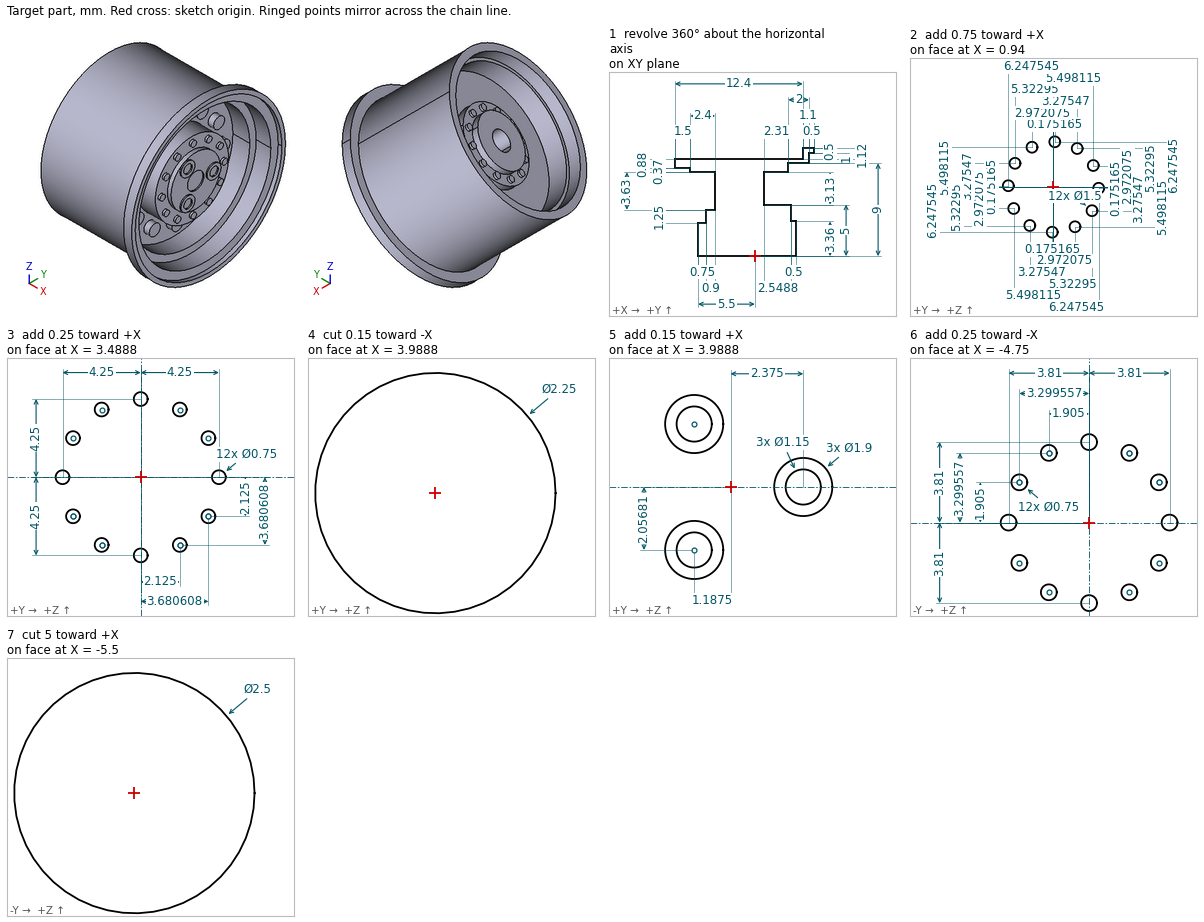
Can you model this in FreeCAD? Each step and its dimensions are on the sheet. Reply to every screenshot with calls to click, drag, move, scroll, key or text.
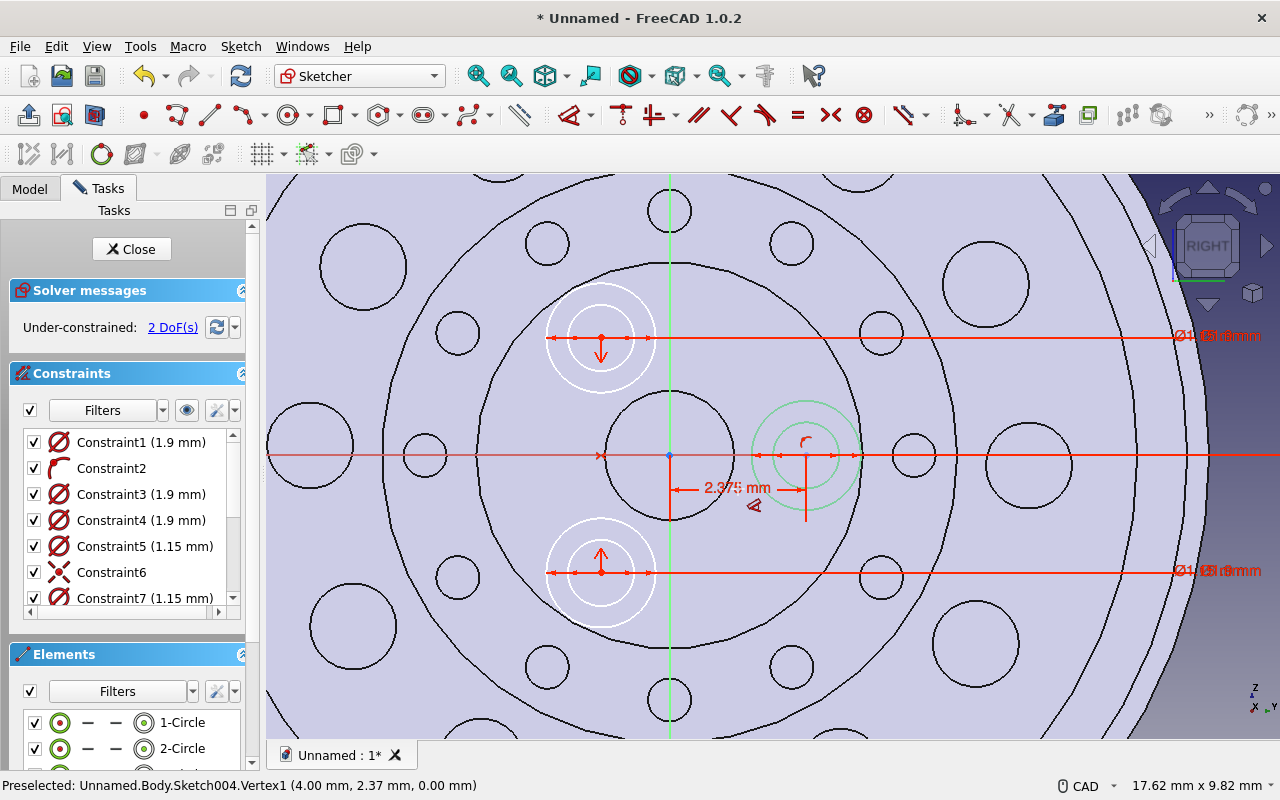
click(601, 573)
click(635, 421)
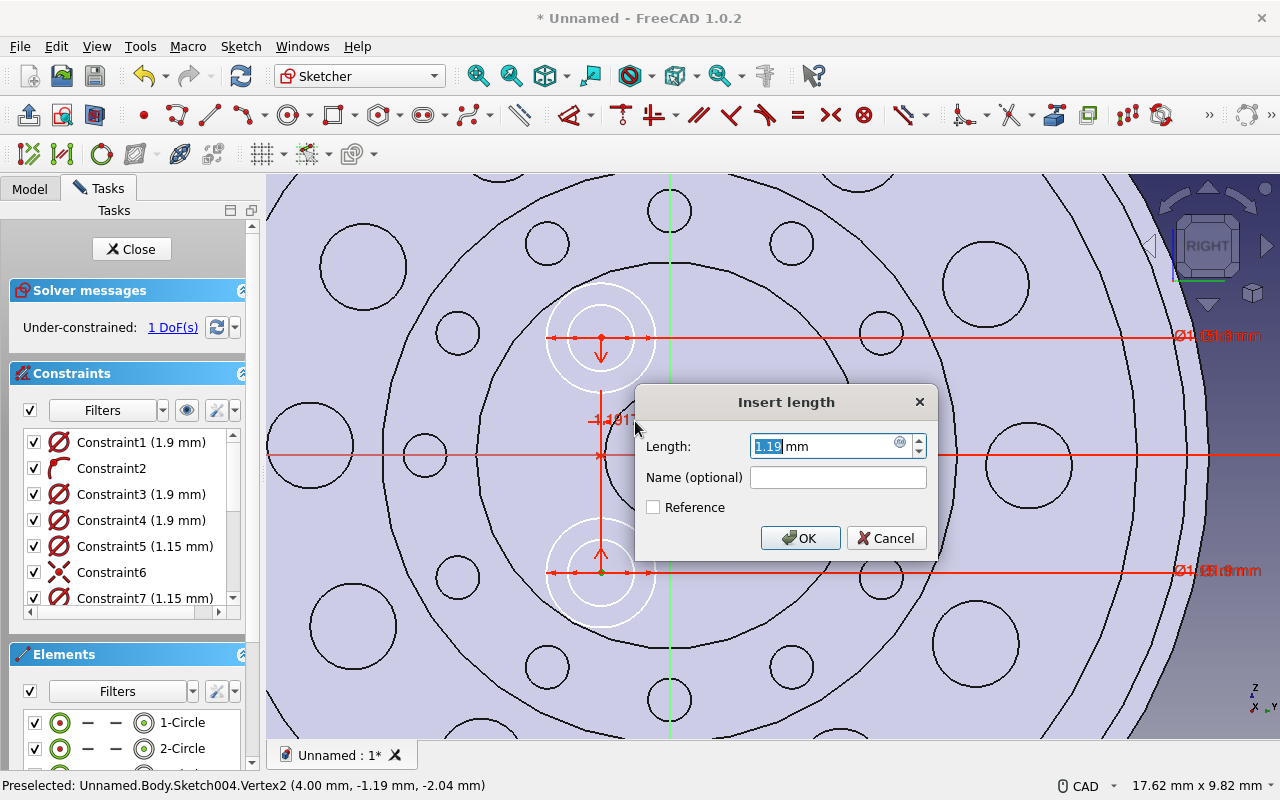
text(1.1875)
key(Return)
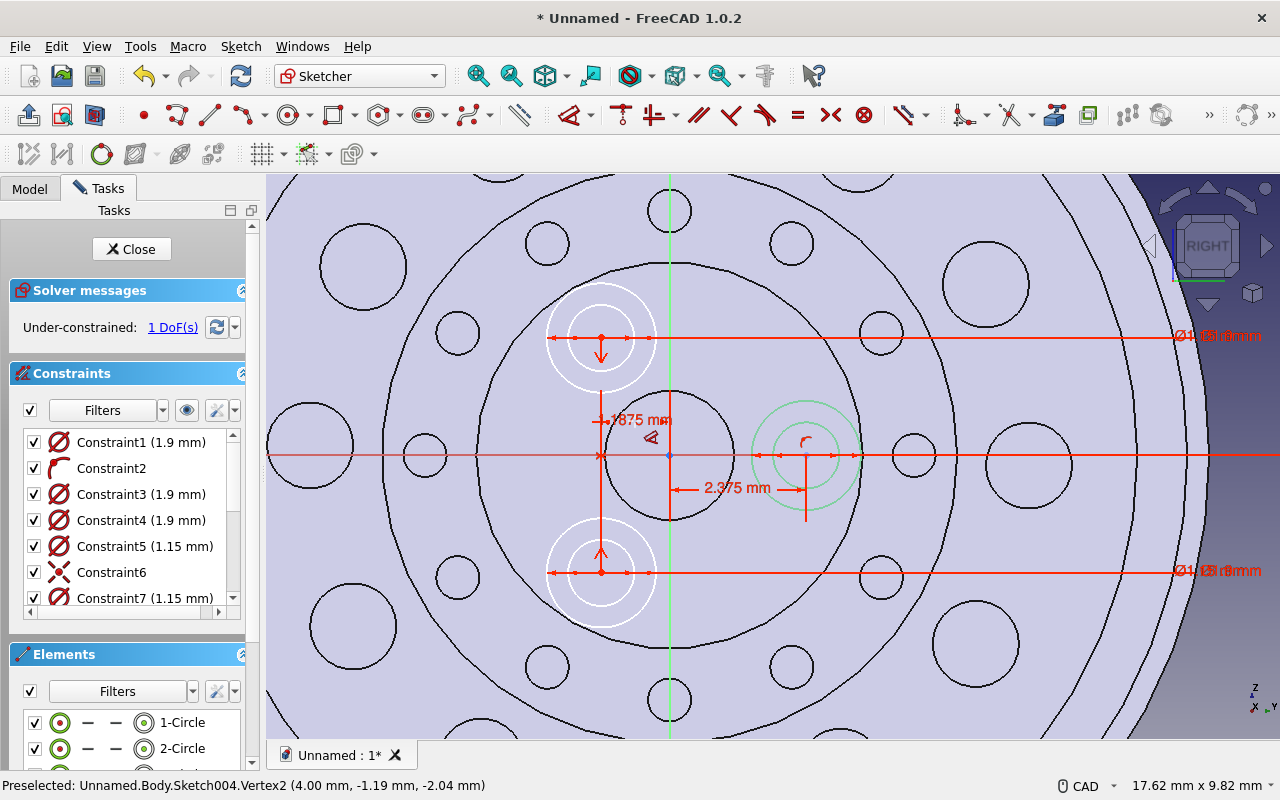
click(601, 573)
click(567, 514)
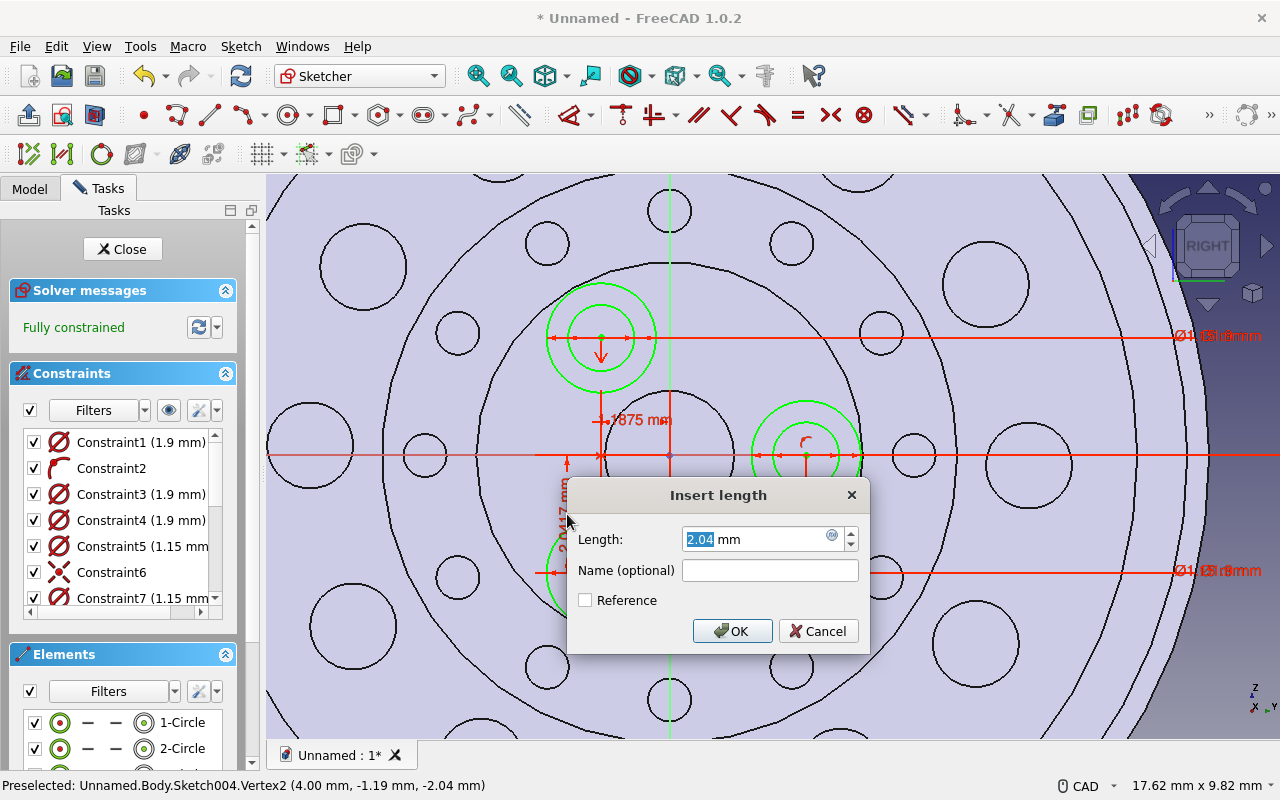
text(2.05681)
key(Return)
key(Escape)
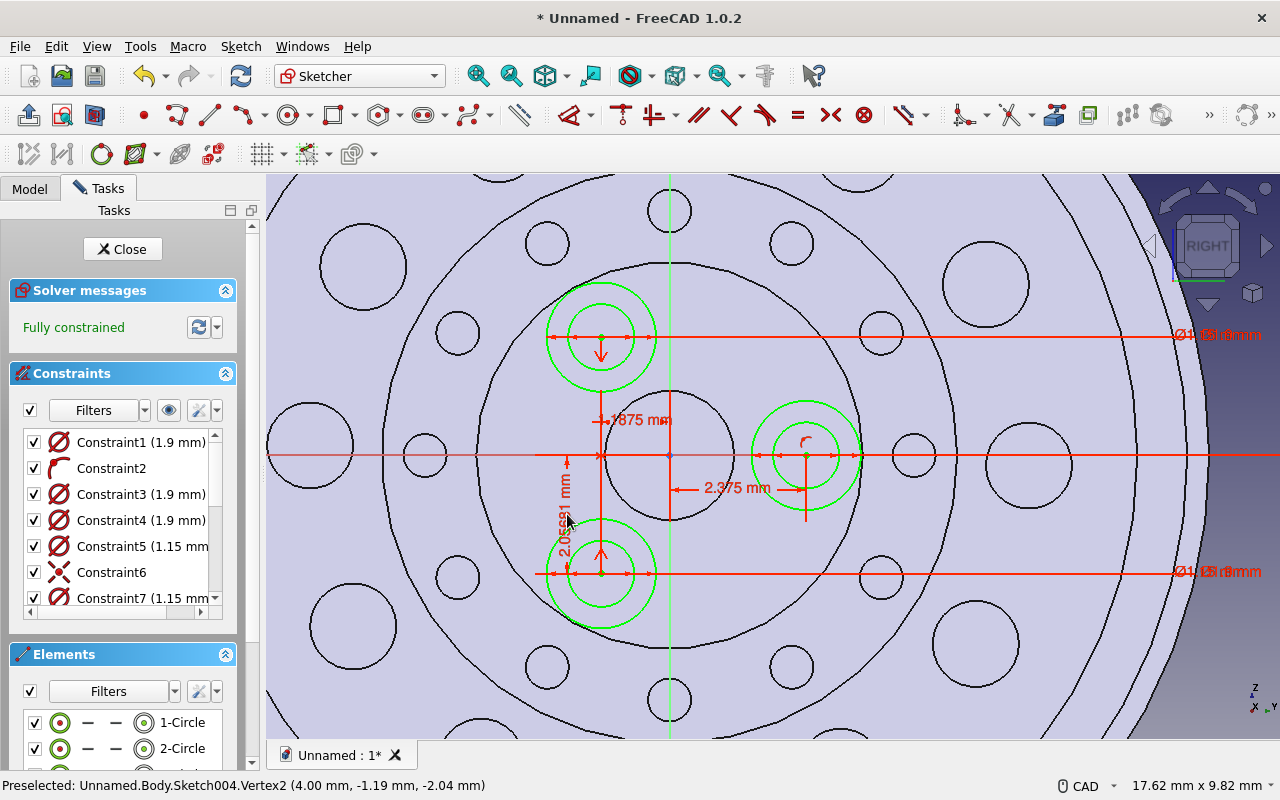
click(123, 249)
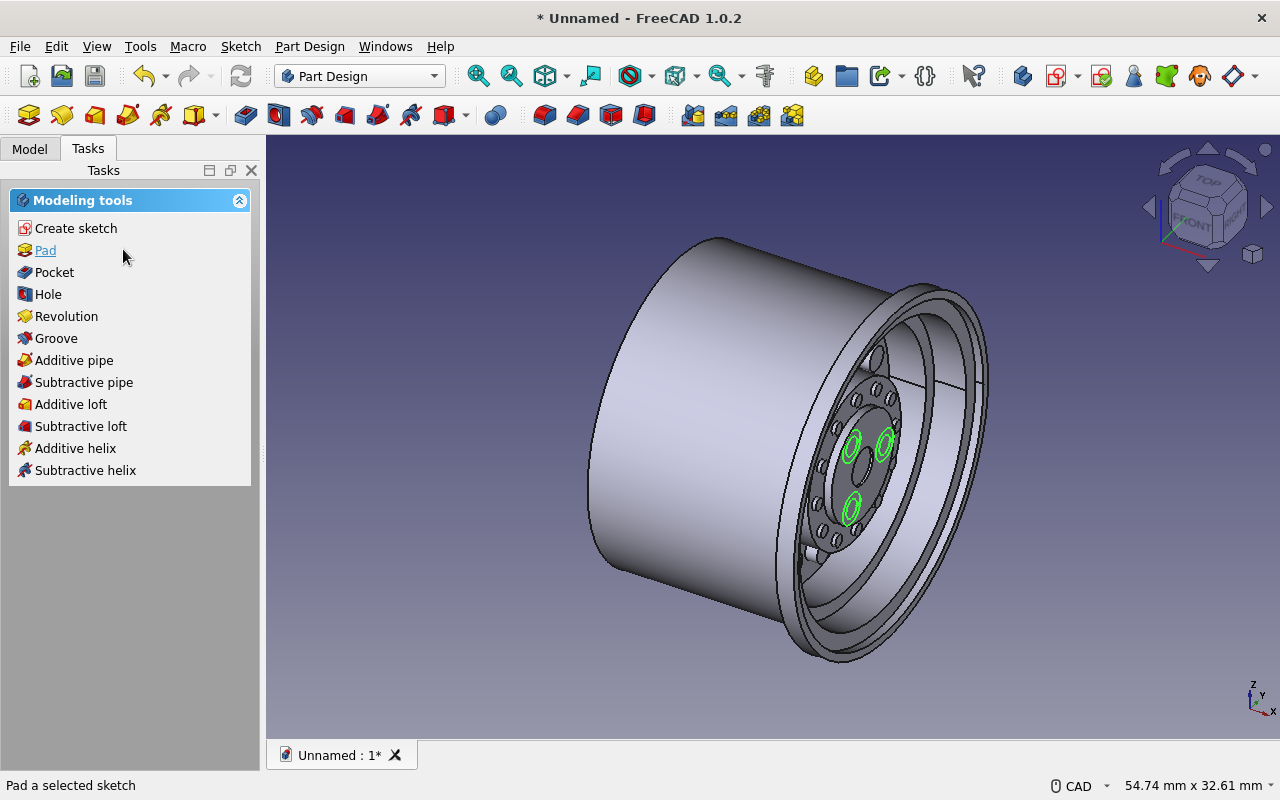
click(29, 116)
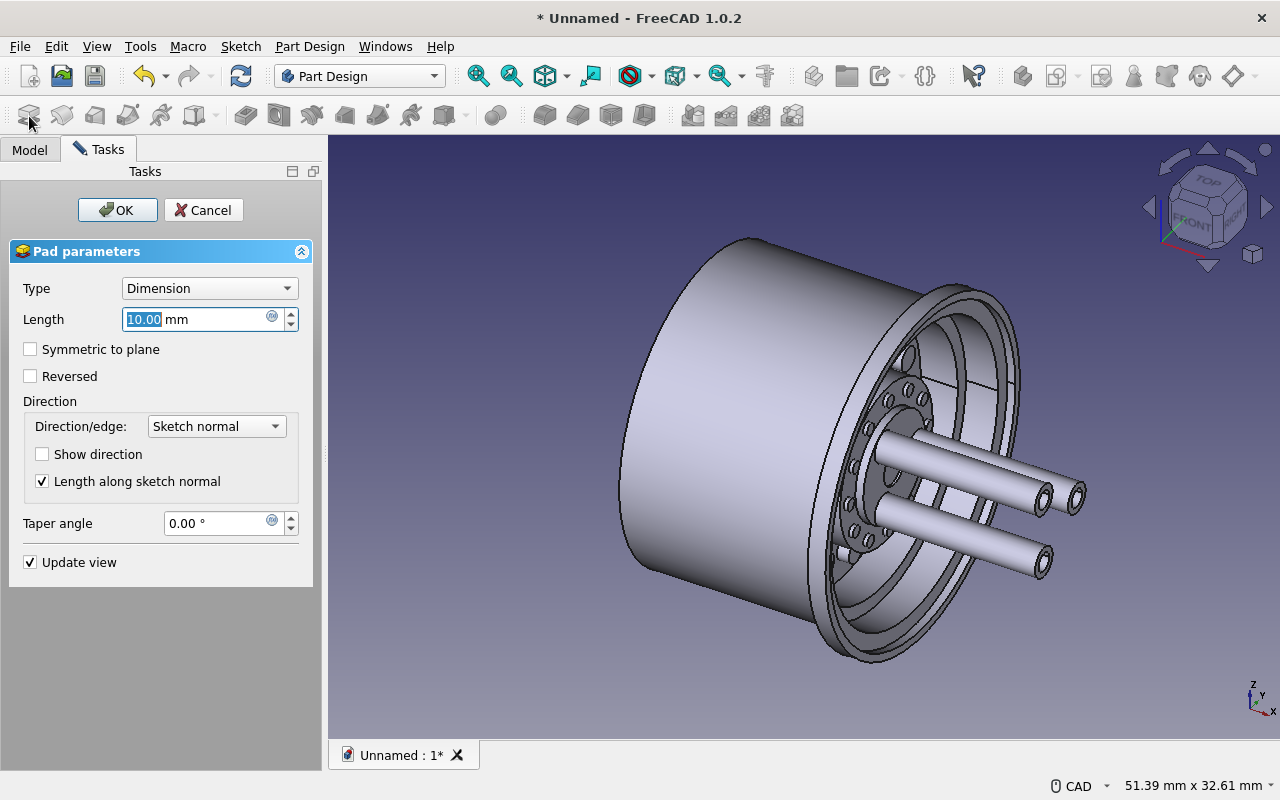
text(0.15)
key(Tab)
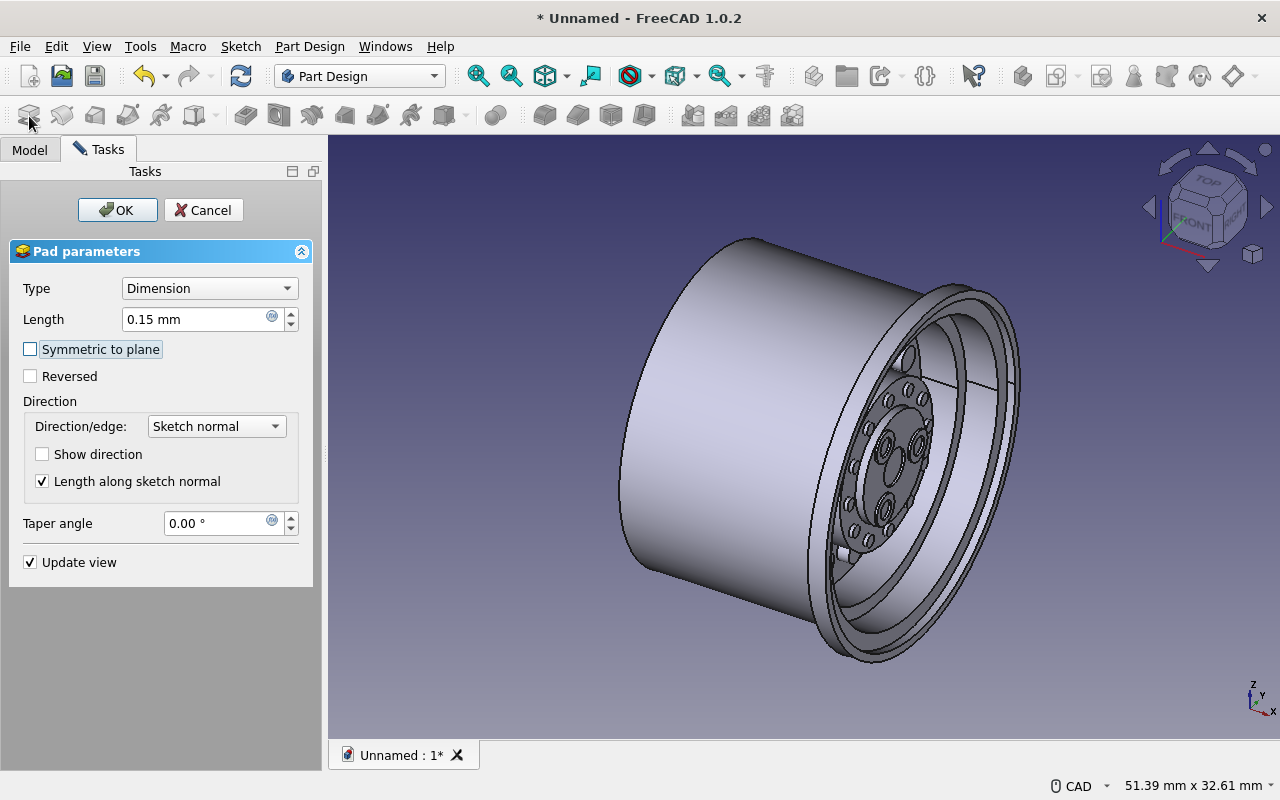
click(118, 210)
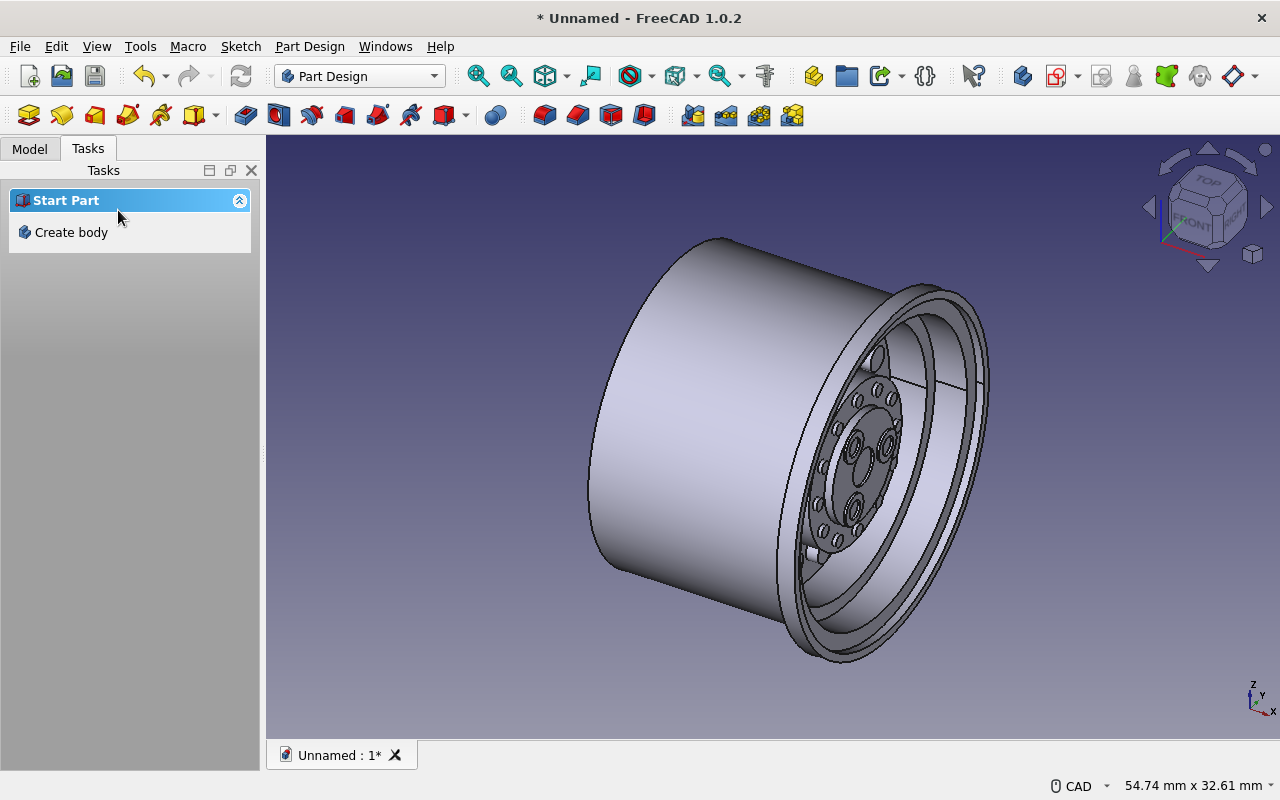
key(6)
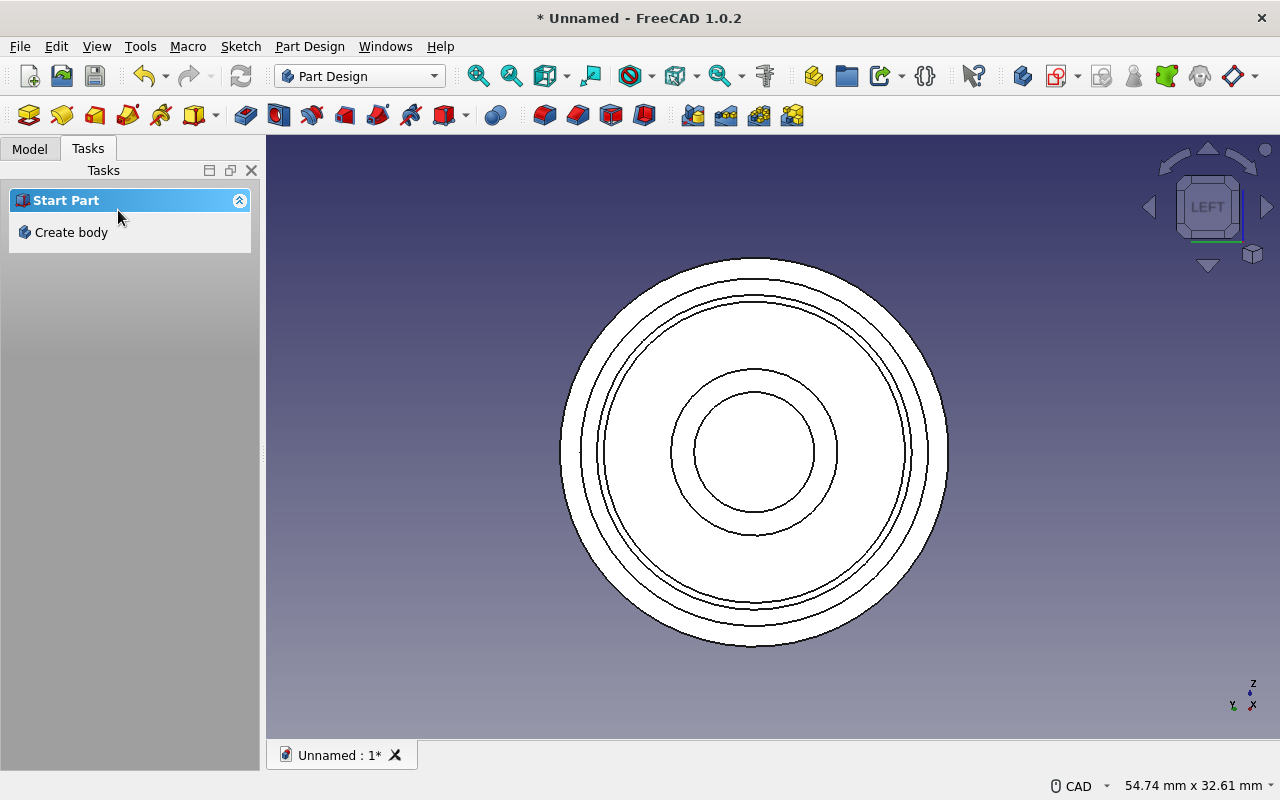
click(683, 451)